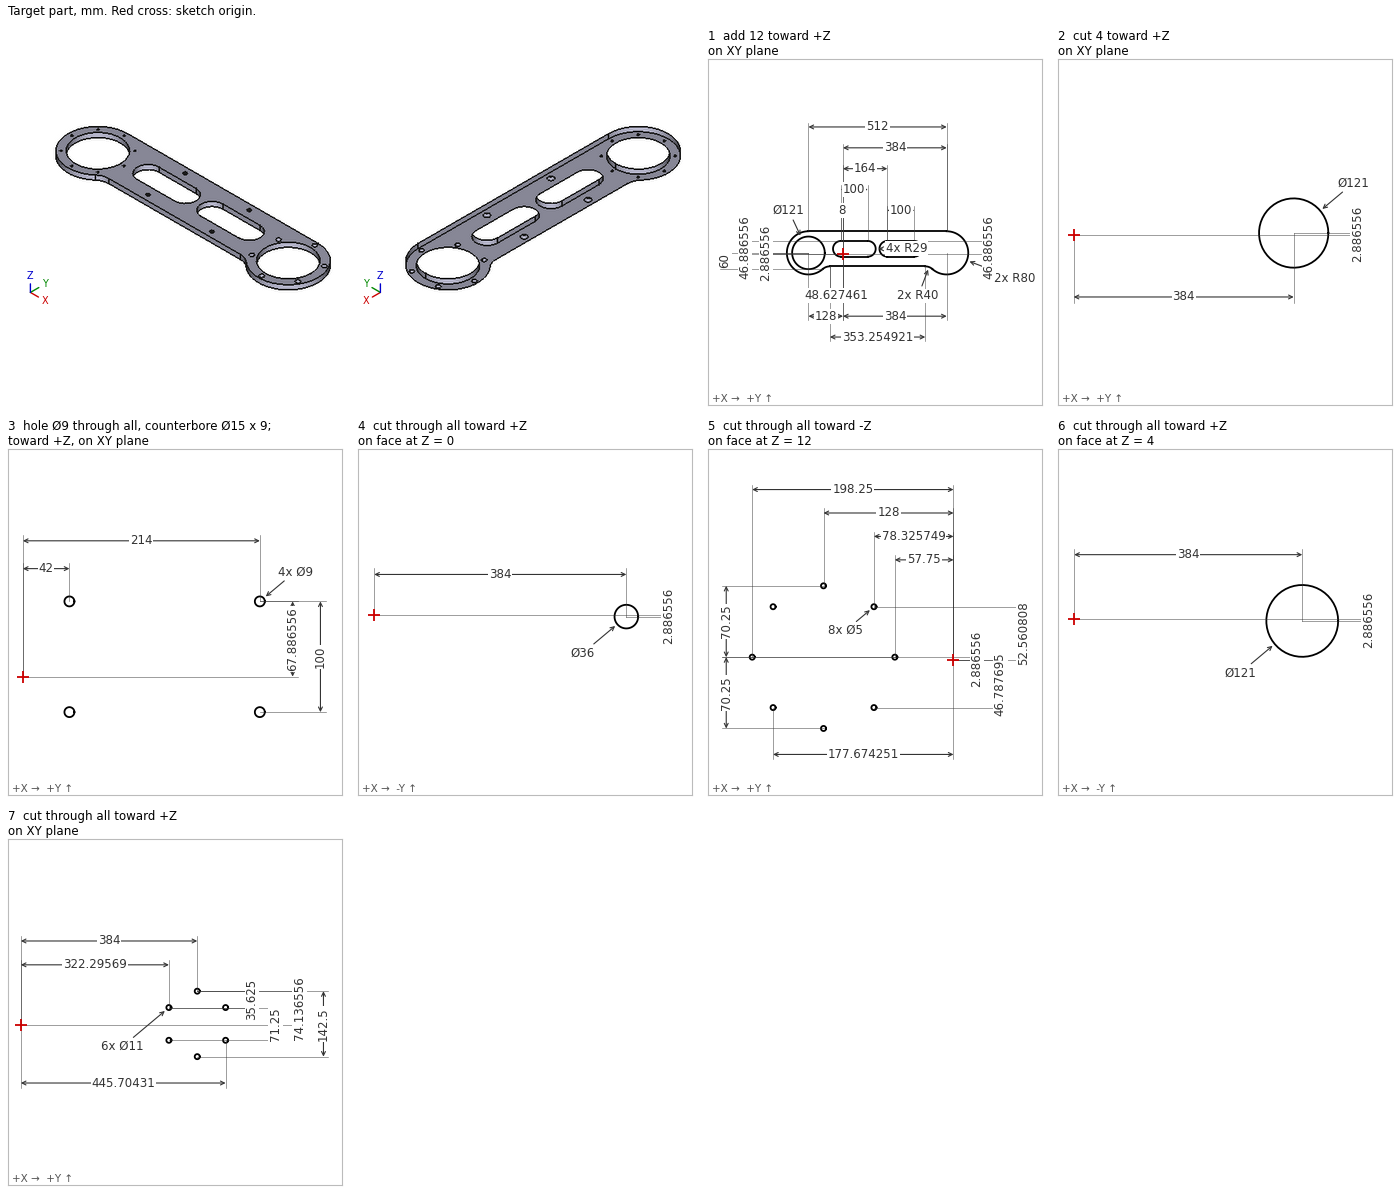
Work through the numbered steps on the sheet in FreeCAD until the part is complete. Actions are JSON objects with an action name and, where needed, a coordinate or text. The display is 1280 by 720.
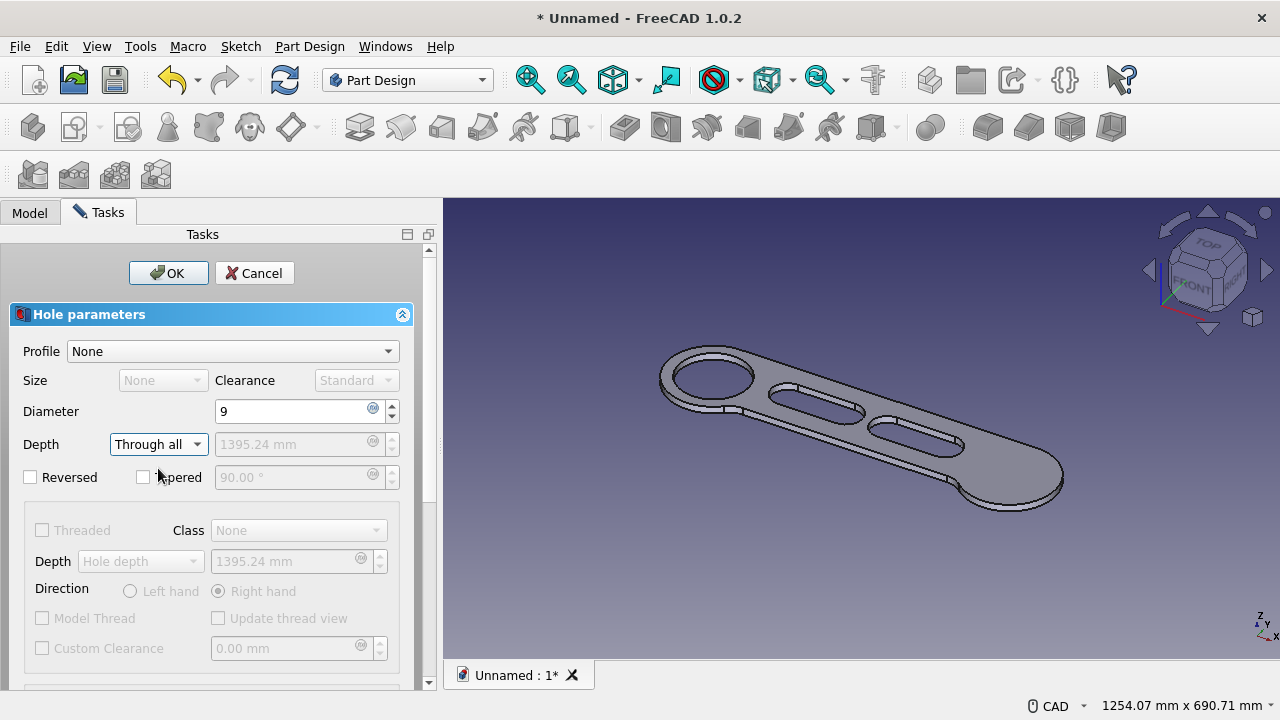
{"action": "left_click", "coordinate": [31, 477]}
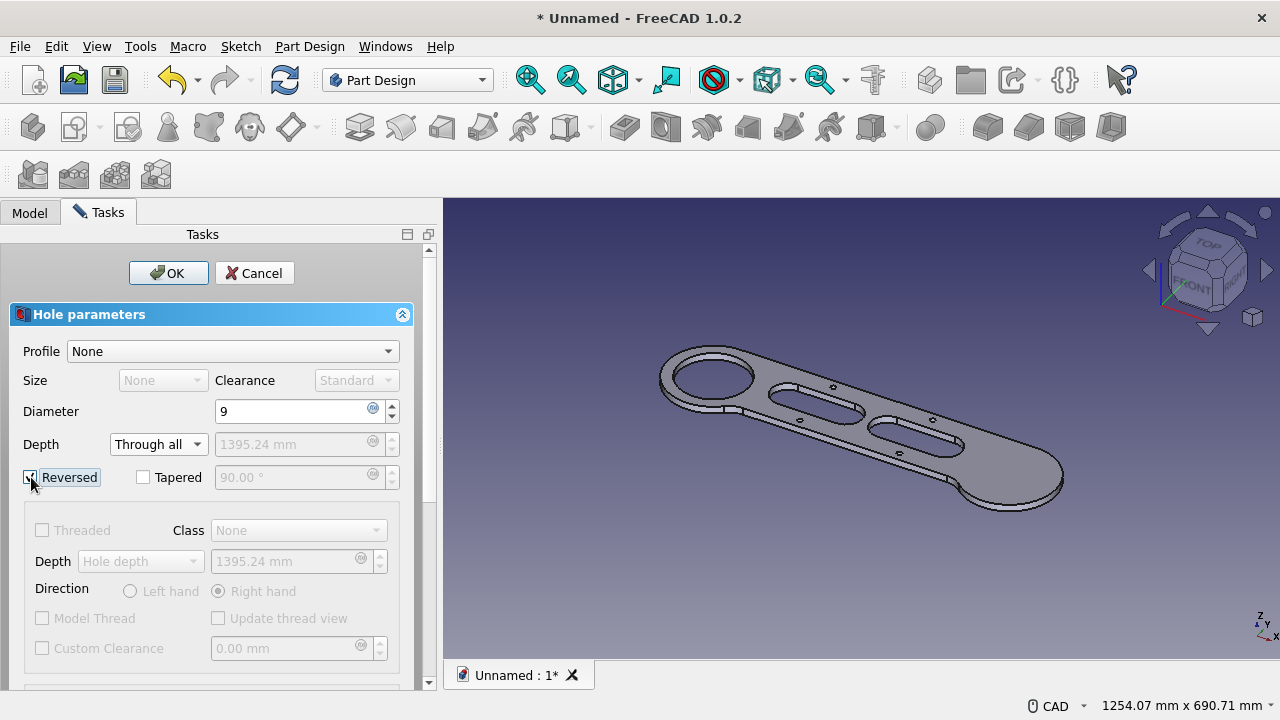
{"action": "scroll", "coordinate": [429, 467], "scroll_direction": "down", "scroll_amount": 2}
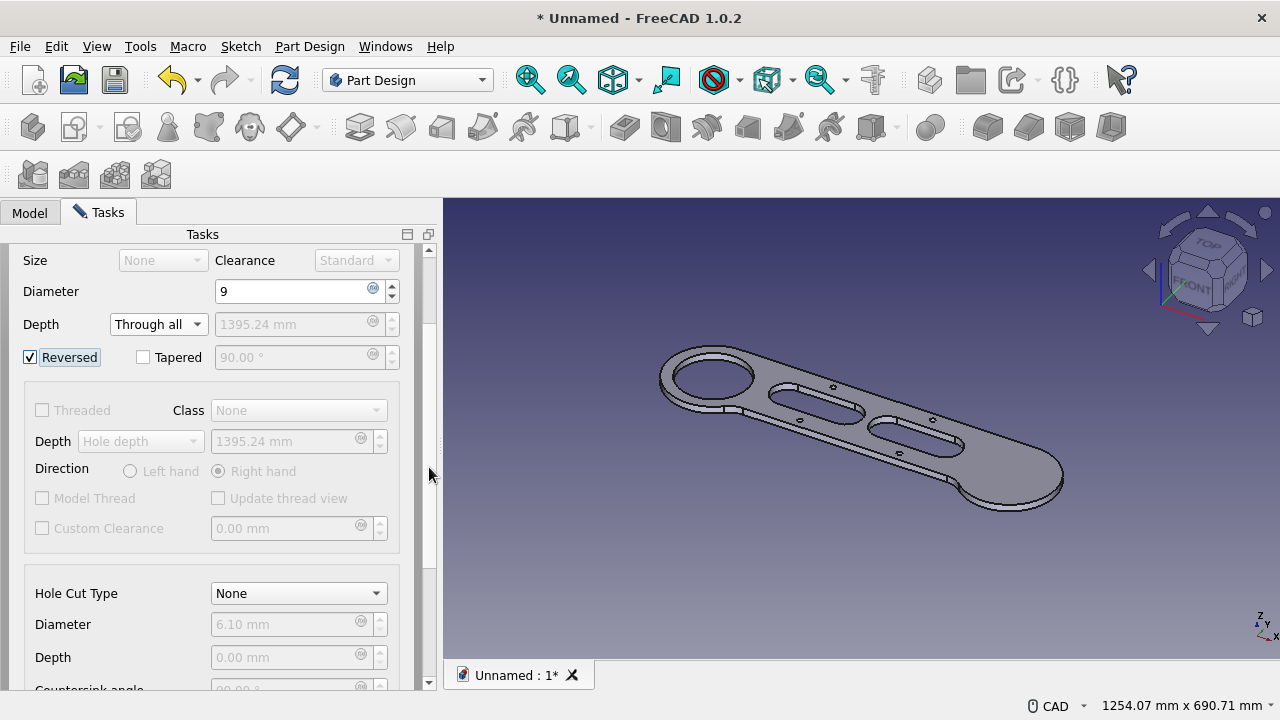
{"action": "left_click", "coordinate": [300, 594]}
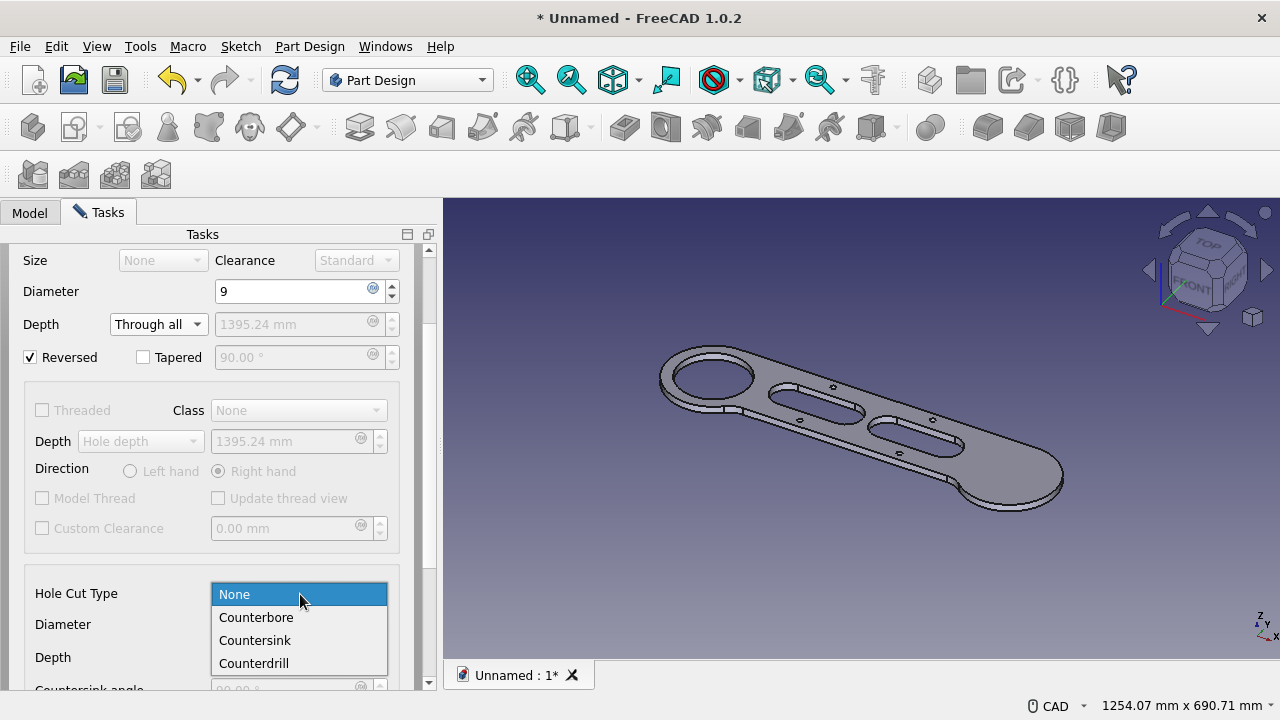
{"action": "left_click", "coordinate": [298, 618]}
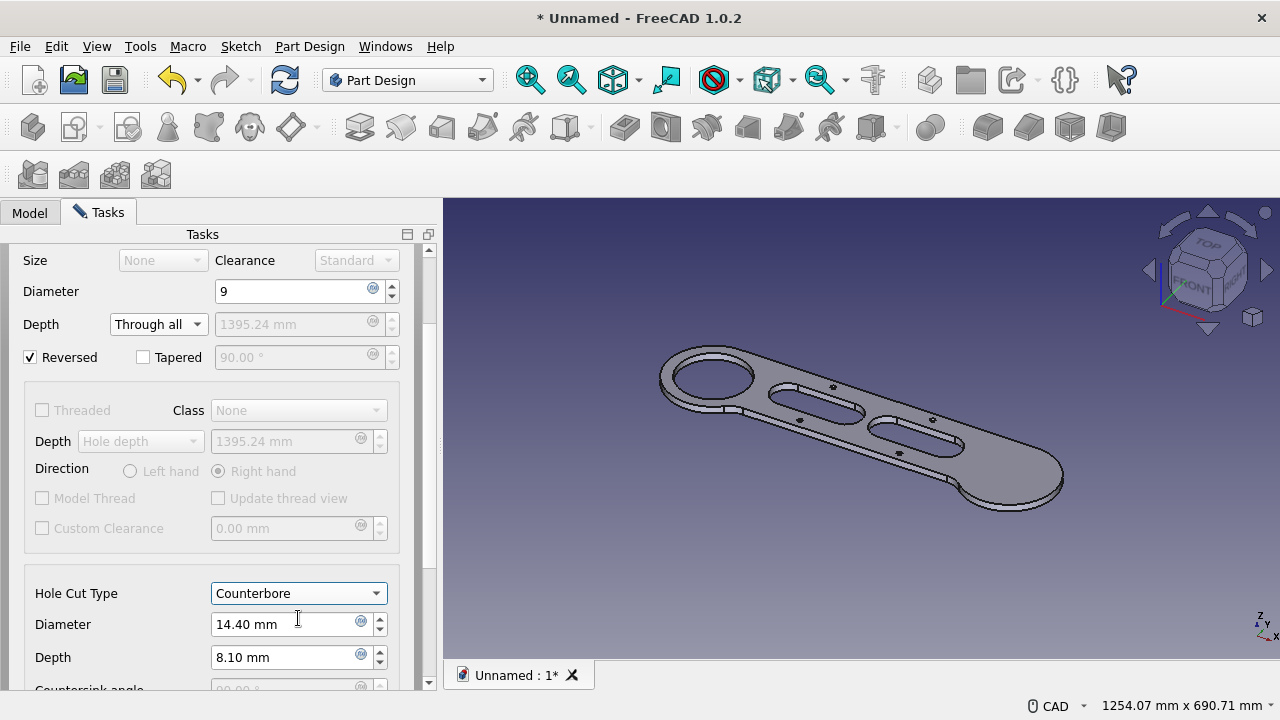
{"action": "triple_click", "coordinate": [292, 624]}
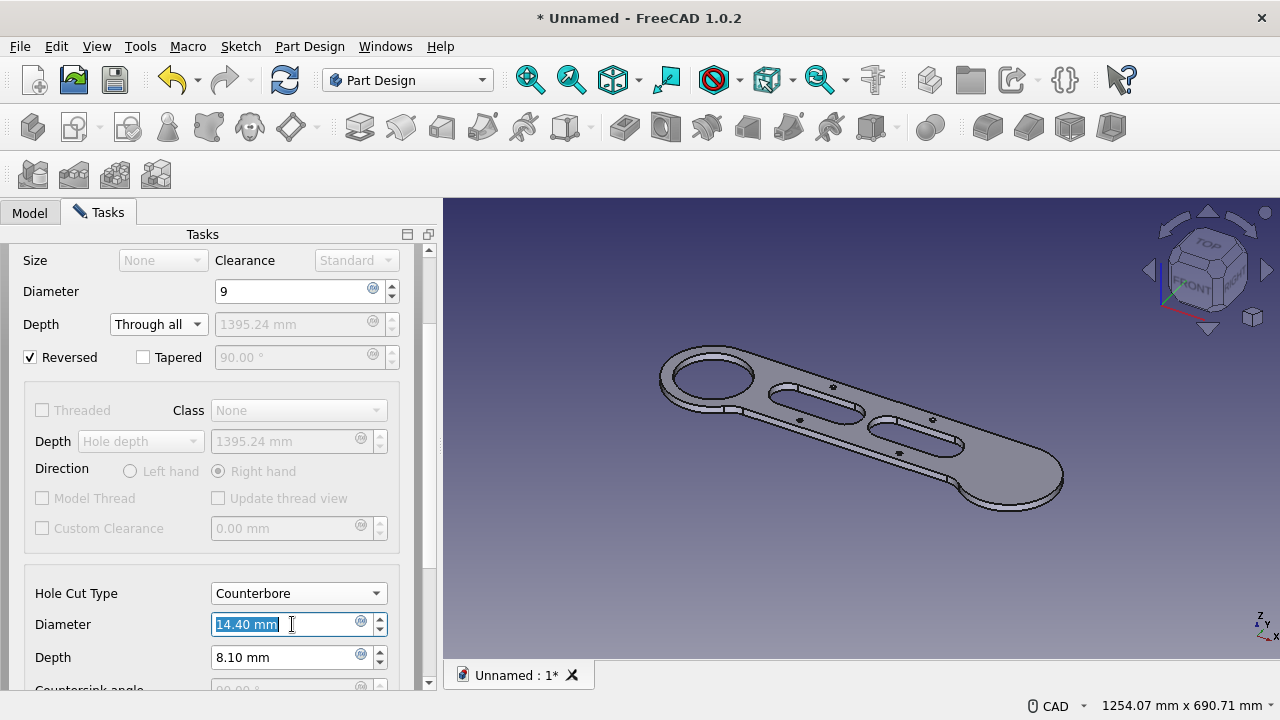
{"action": "type", "text": "15"}
{"action": "key", "text": "Tab"}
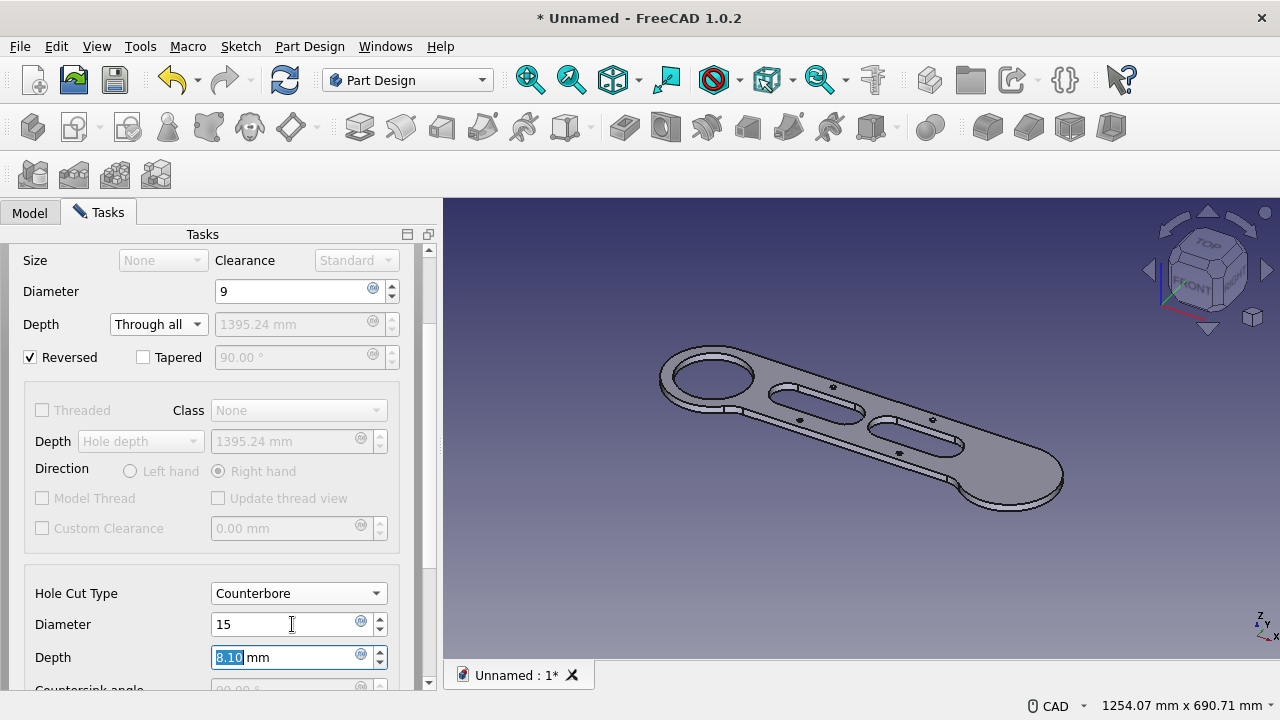
{"action": "type", "text": "9"}
{"action": "key", "text": "Tab"}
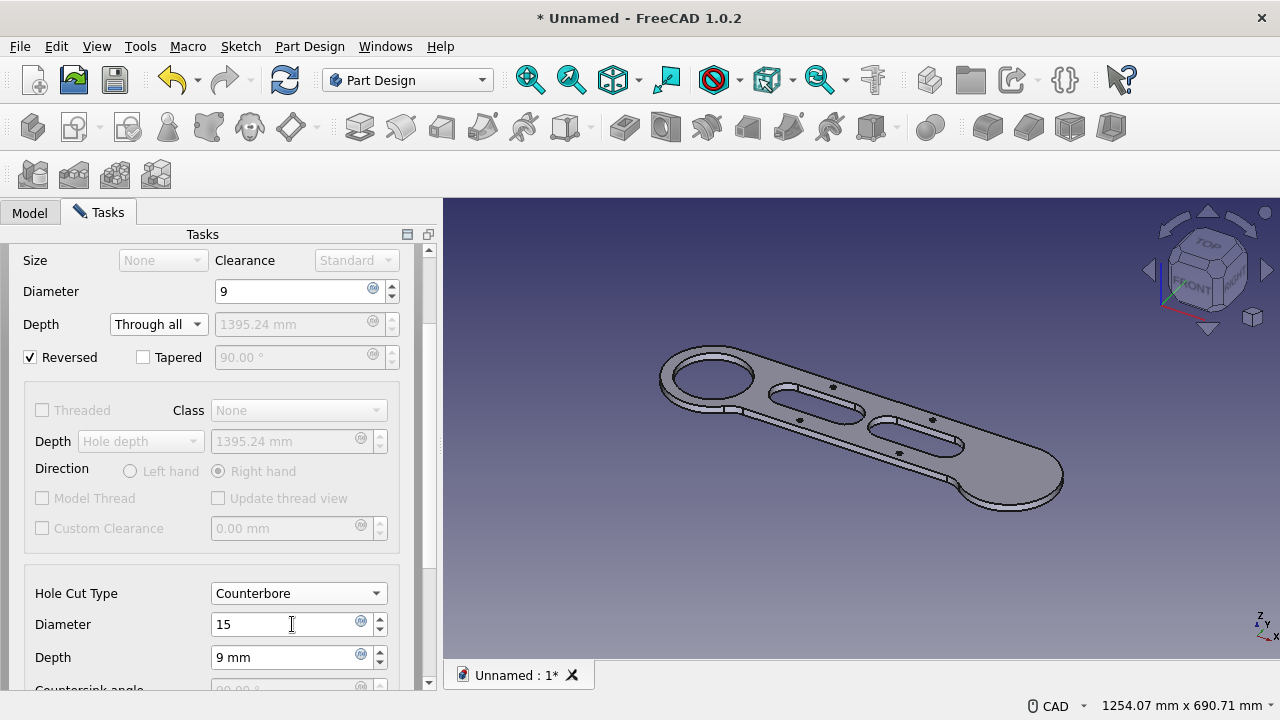
{"action": "scroll", "coordinate": [429, 467], "scroll_direction": "up", "scroll_amount": 3}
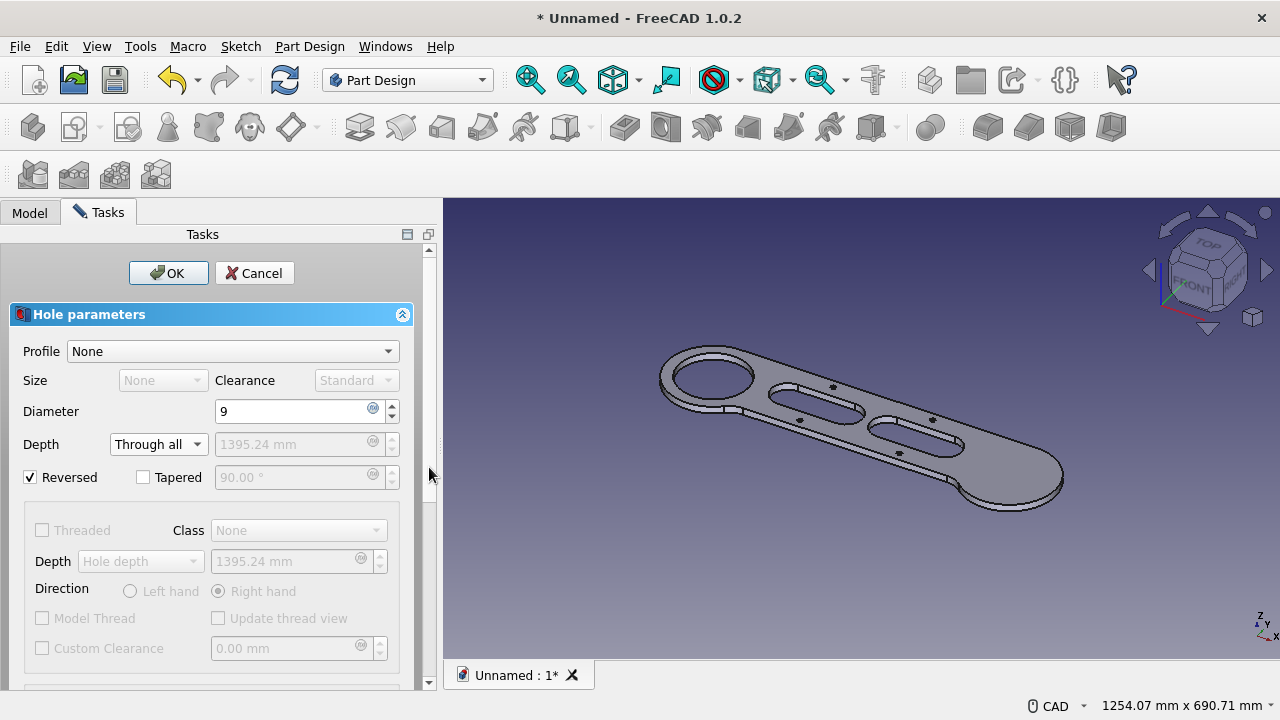
{"action": "left_click", "coordinate": [169, 273]}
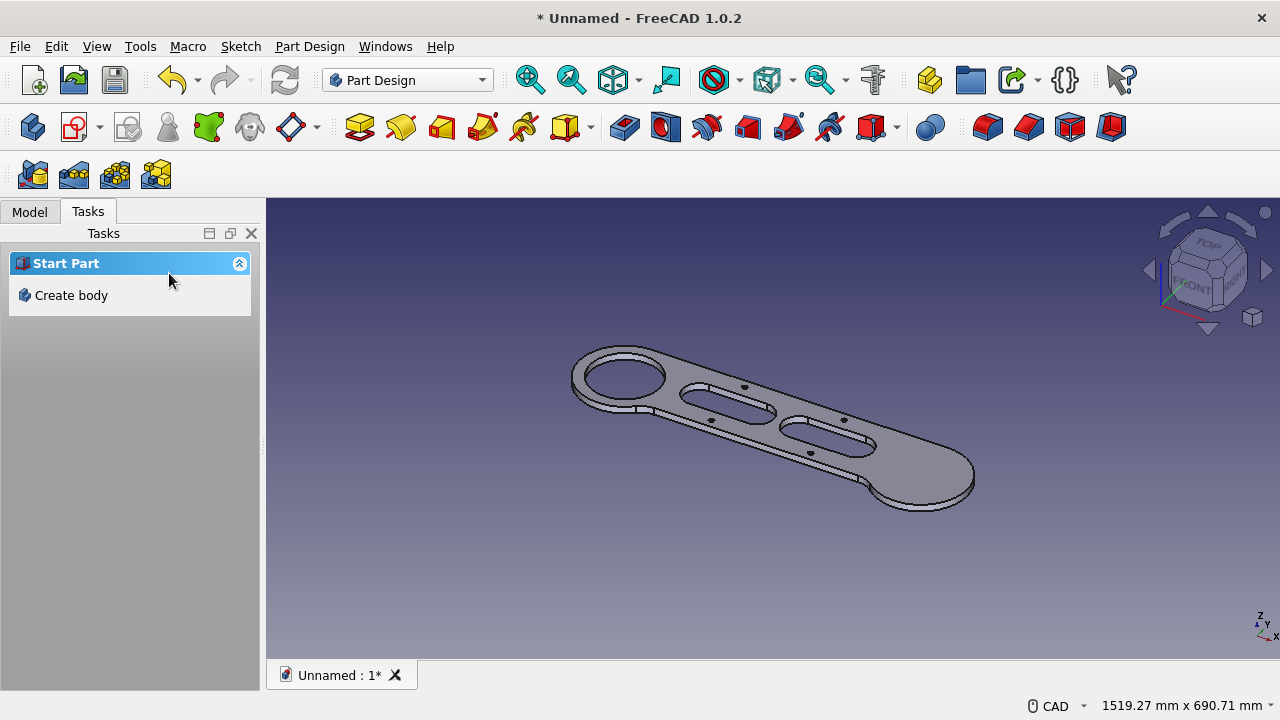
{"action": "left_click", "coordinate": [531, 80]}